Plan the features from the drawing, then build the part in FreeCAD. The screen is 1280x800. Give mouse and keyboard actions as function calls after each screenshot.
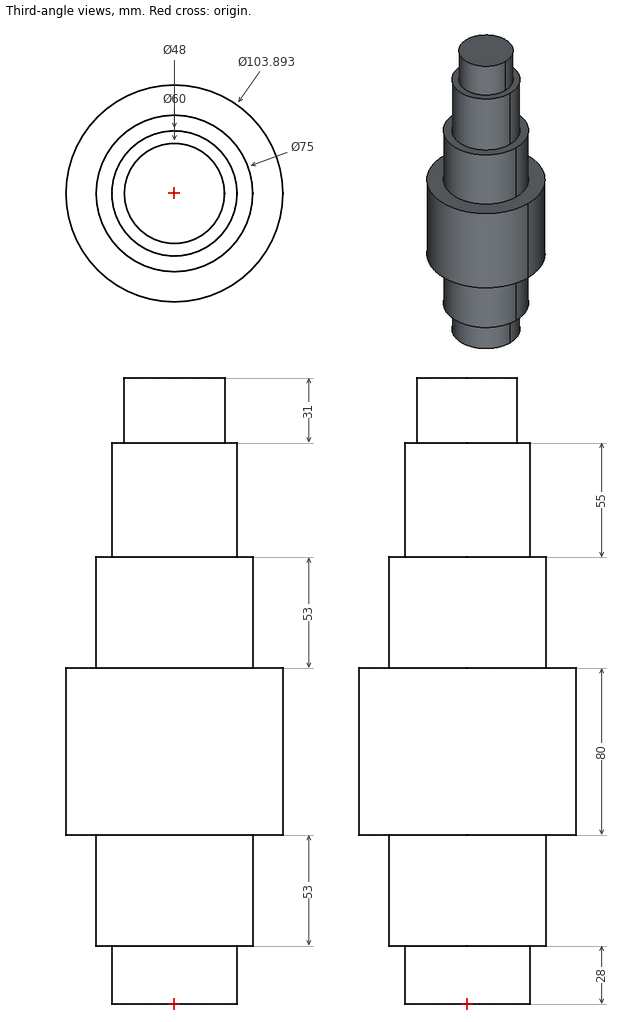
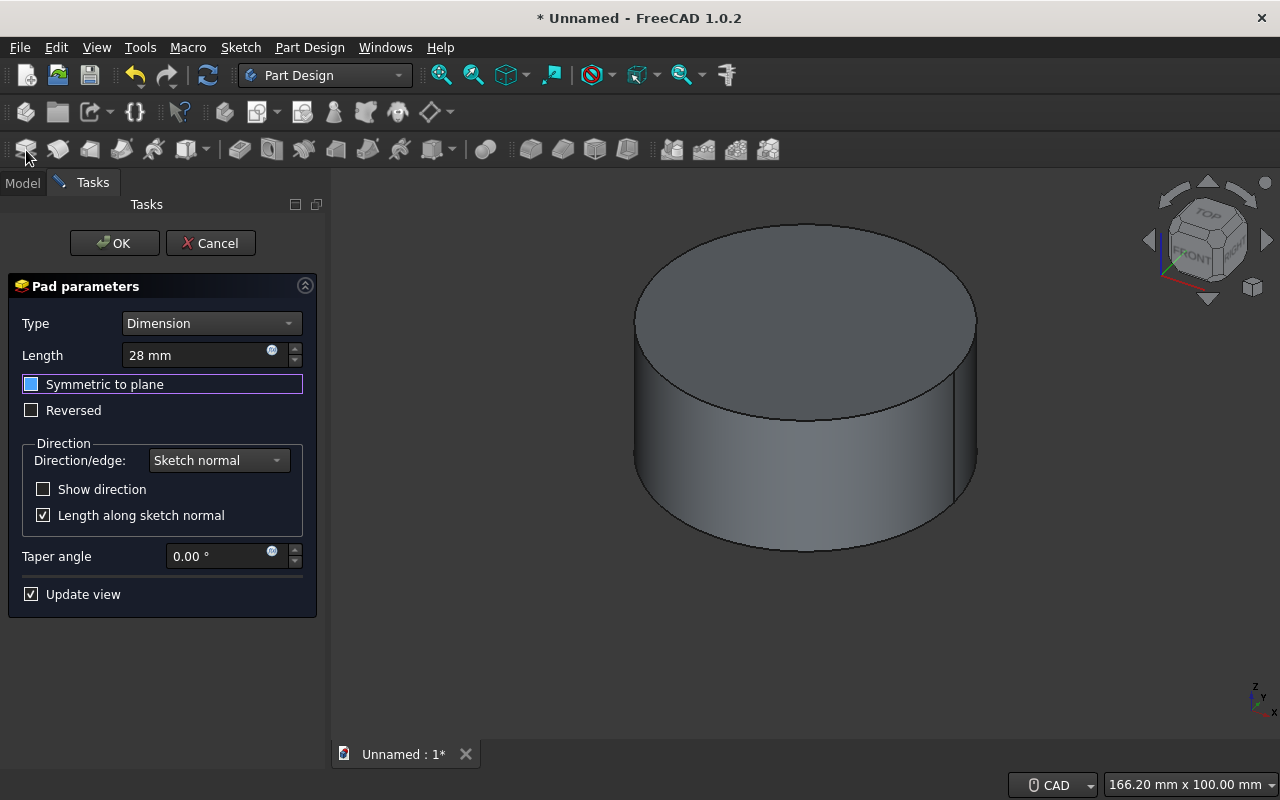
click(115, 243)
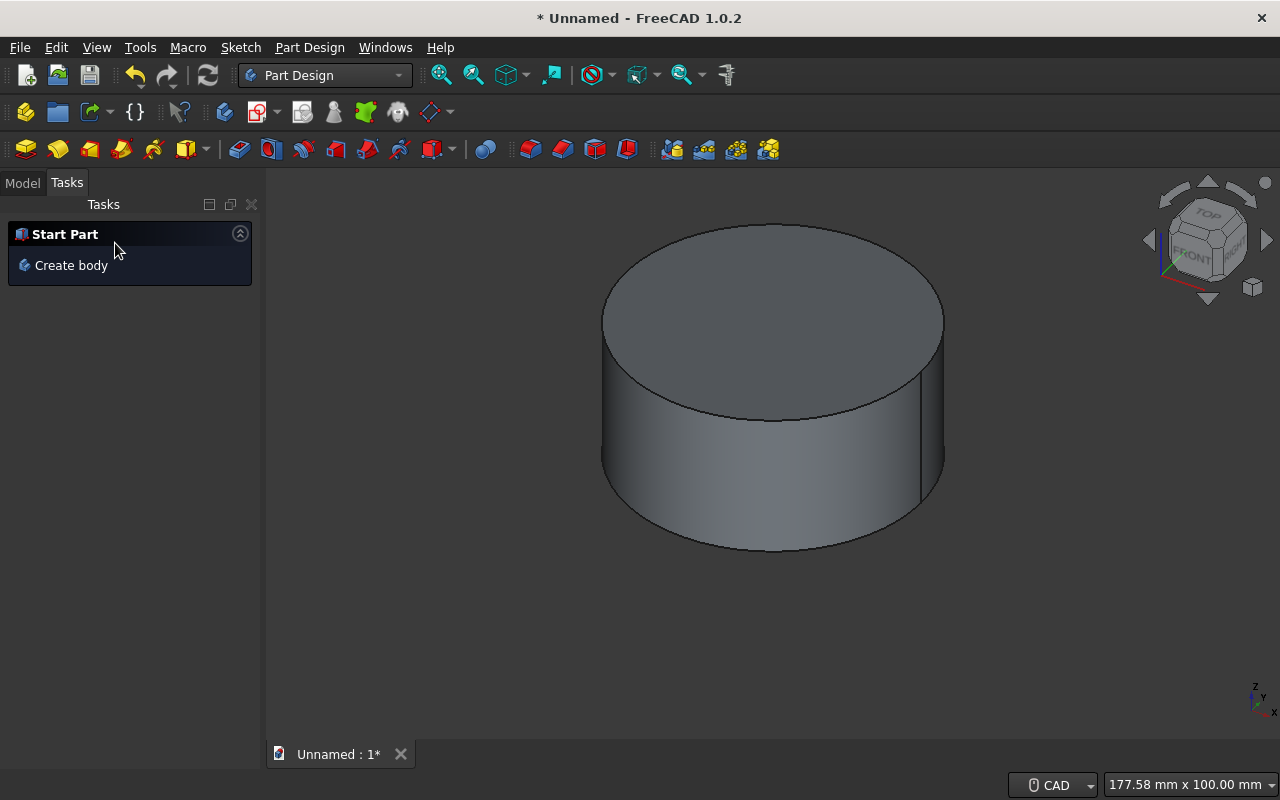
click(773, 322)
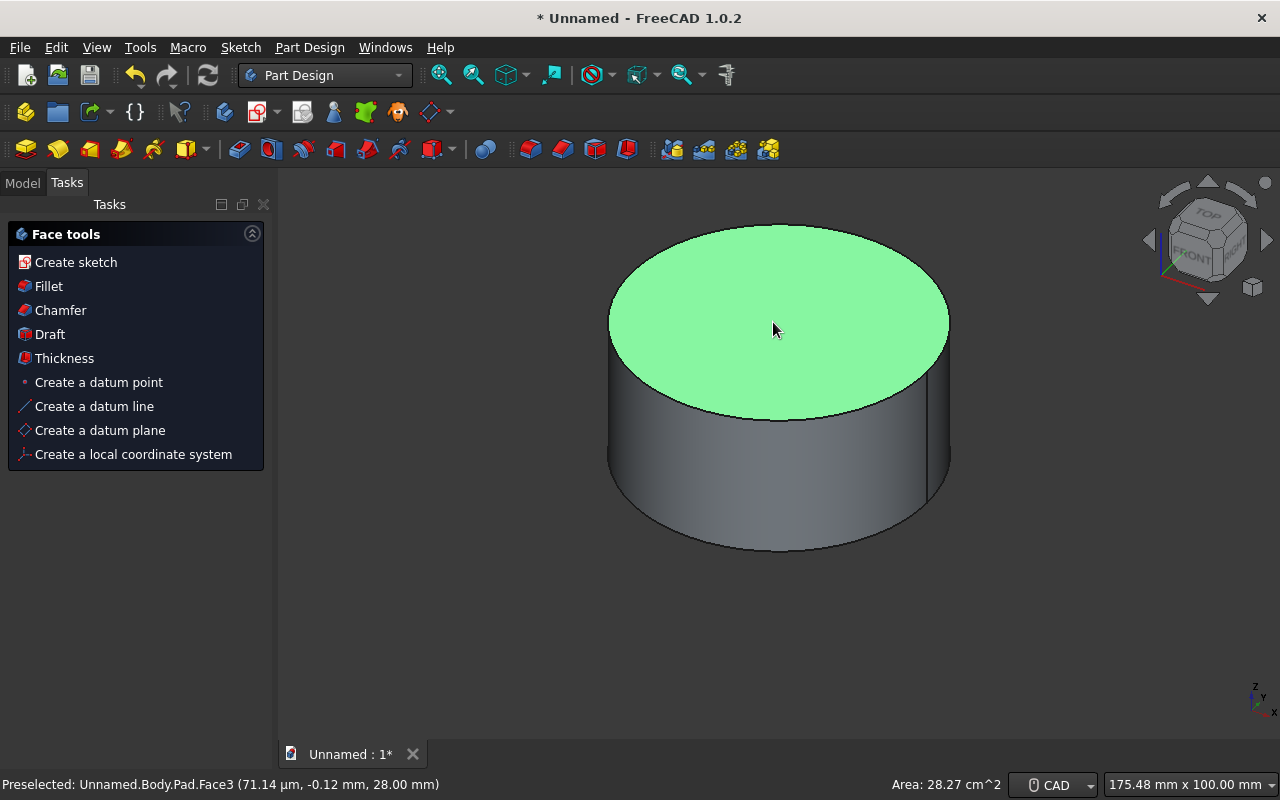
click(258, 112)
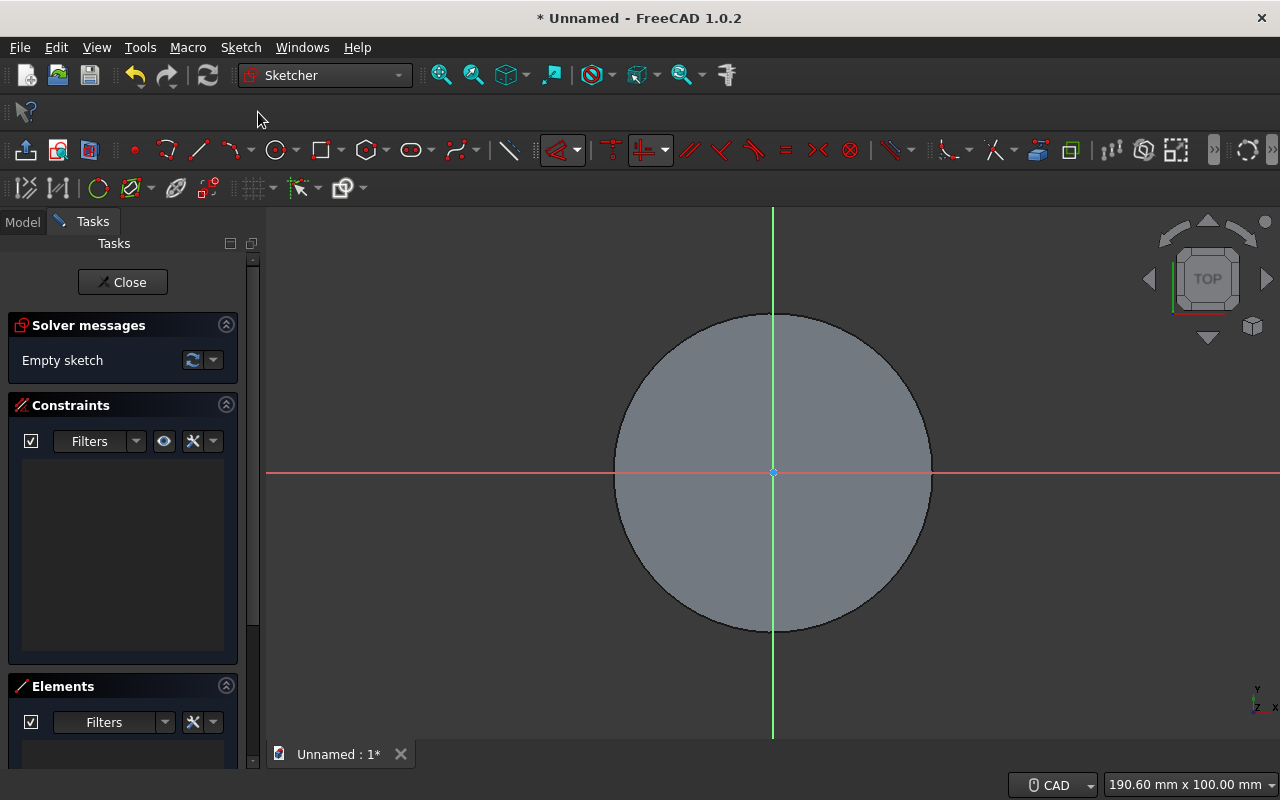
click(276, 150)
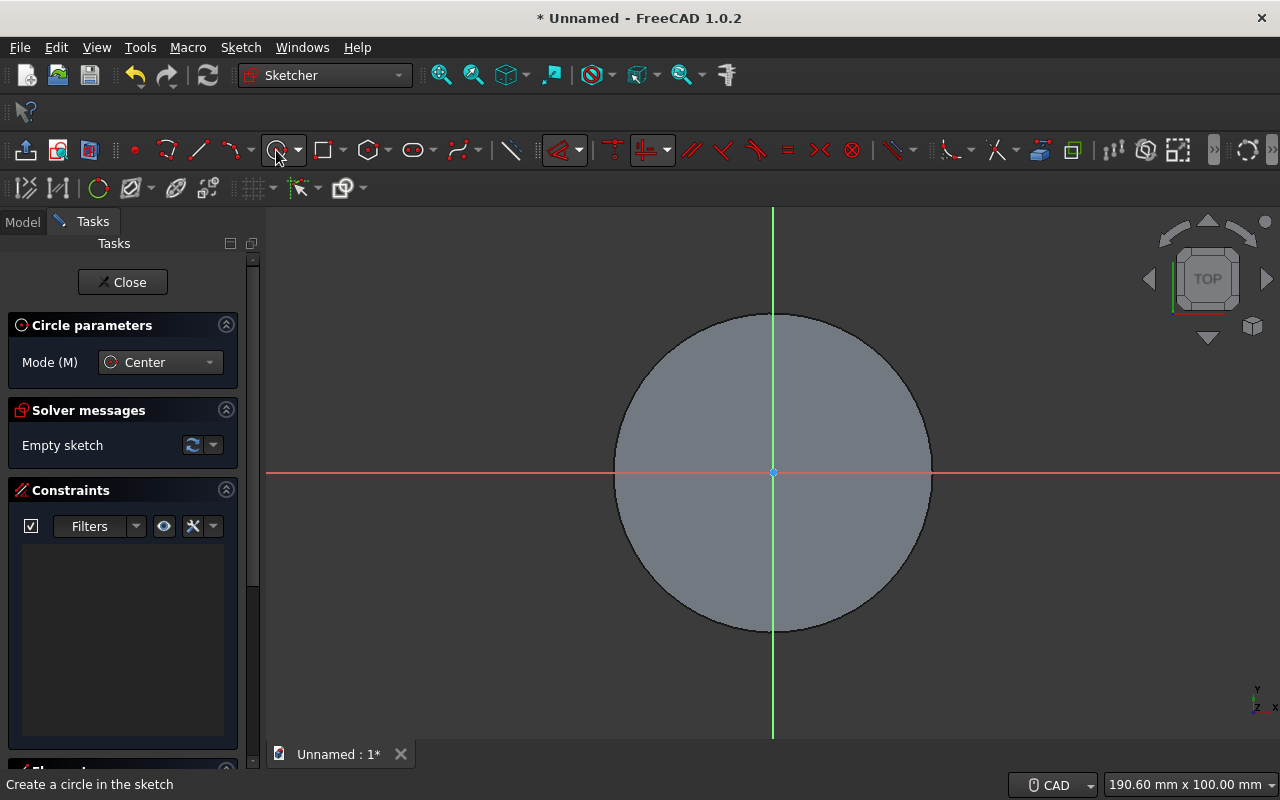
click(773, 473)
move(914, 332)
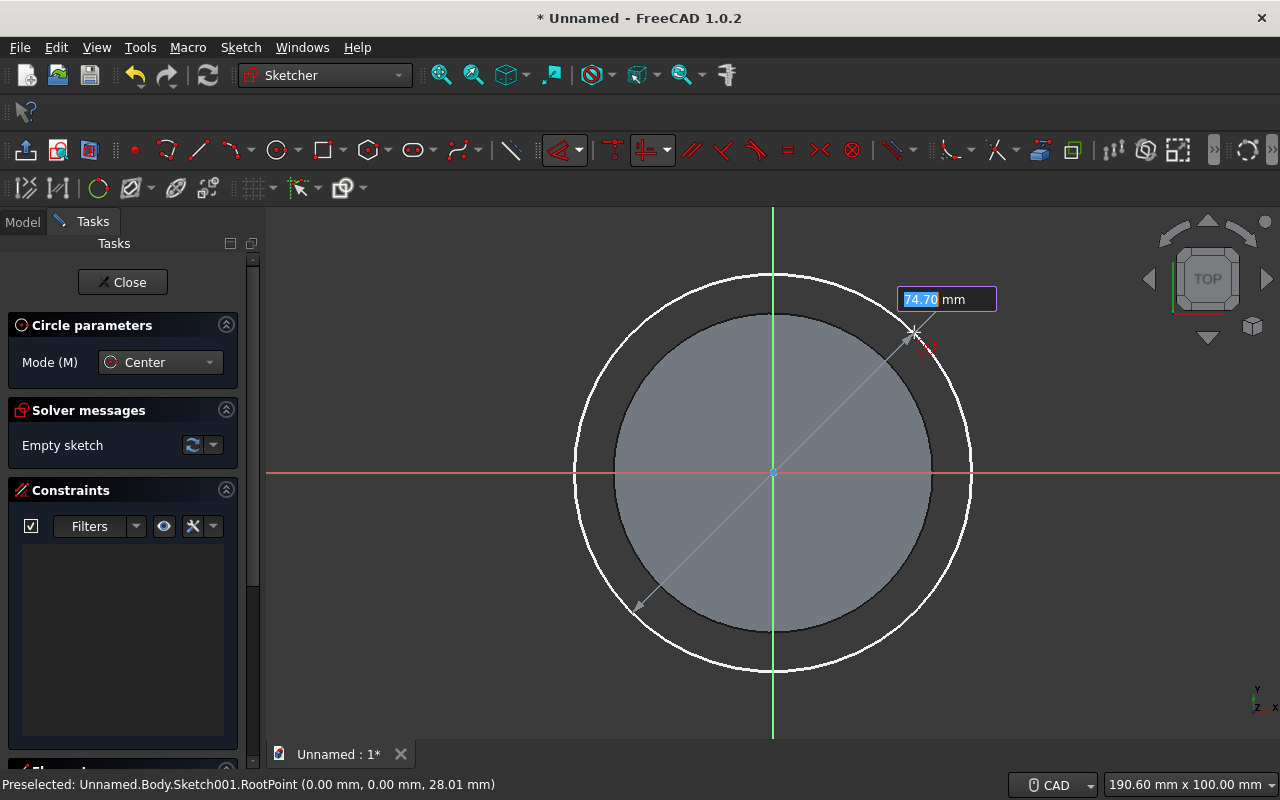
text(75)
key(Return)
key(Escape)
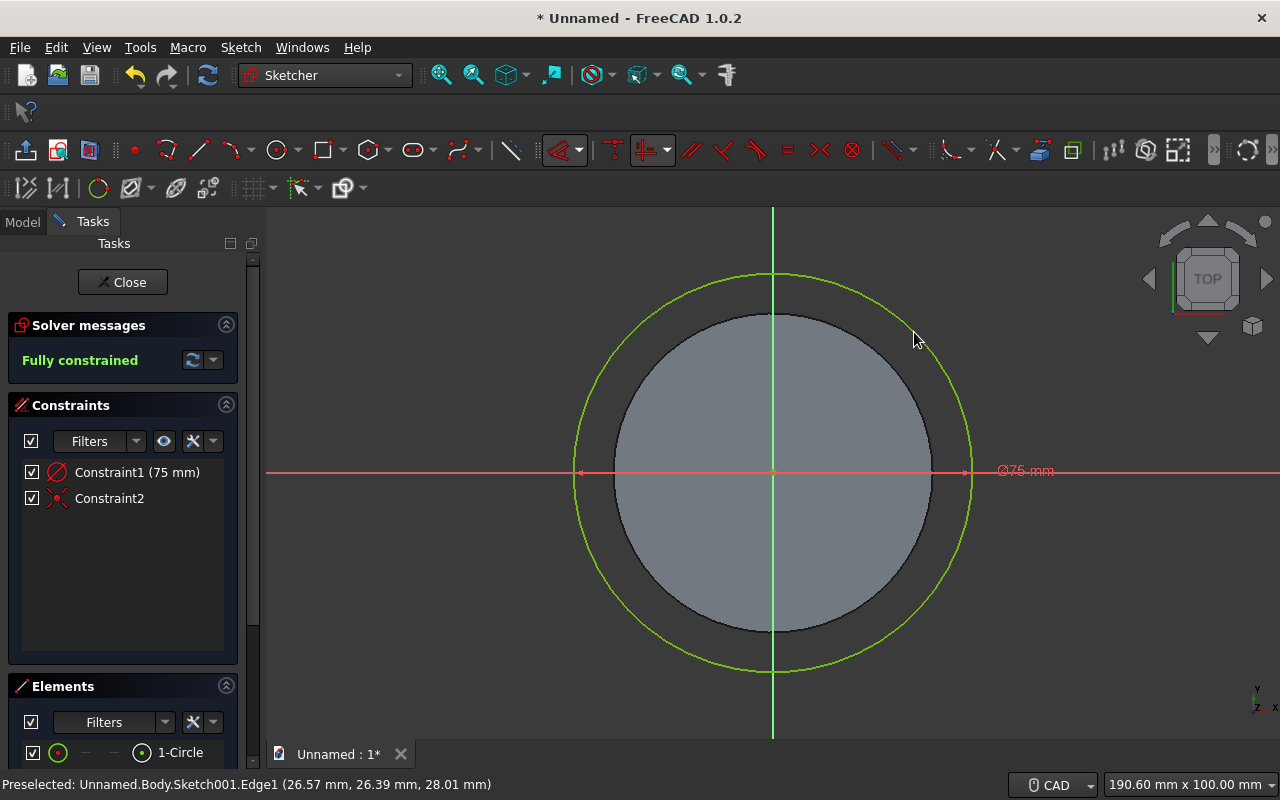
click(123, 282)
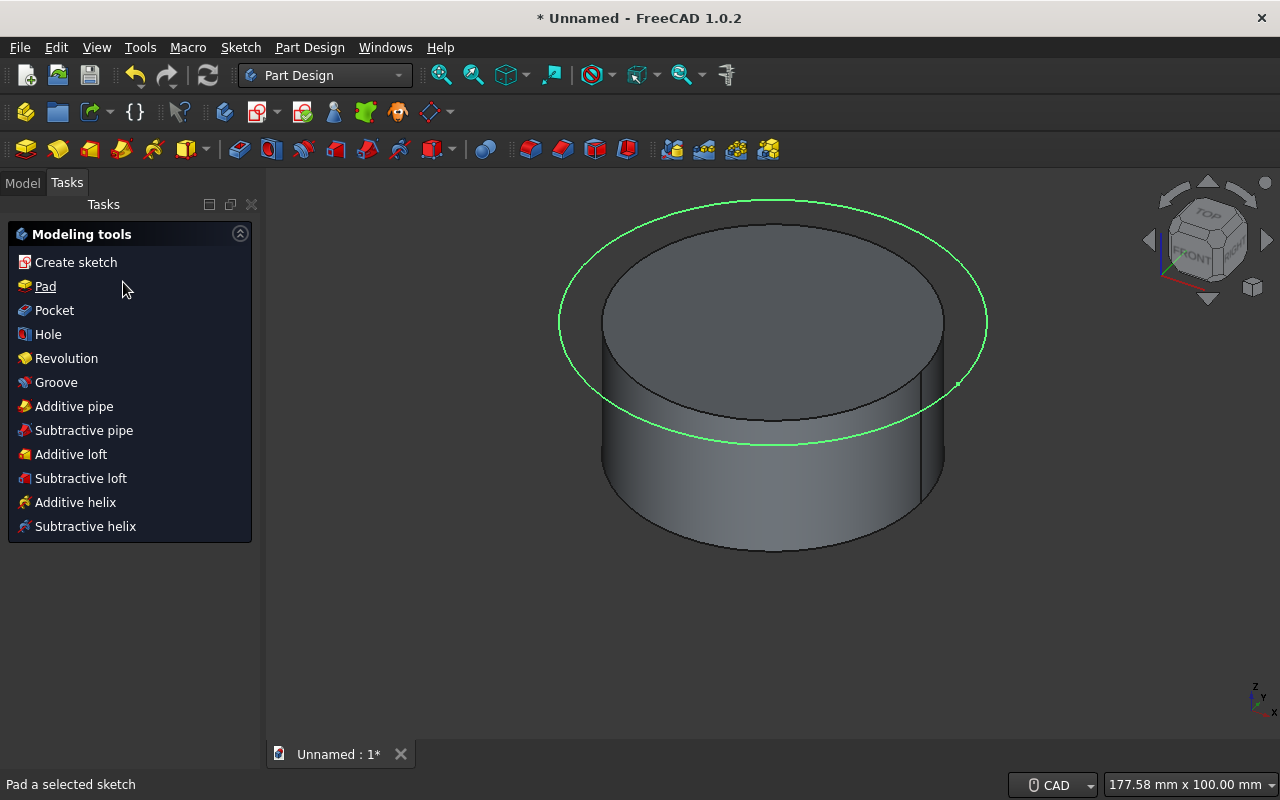
click(26, 150)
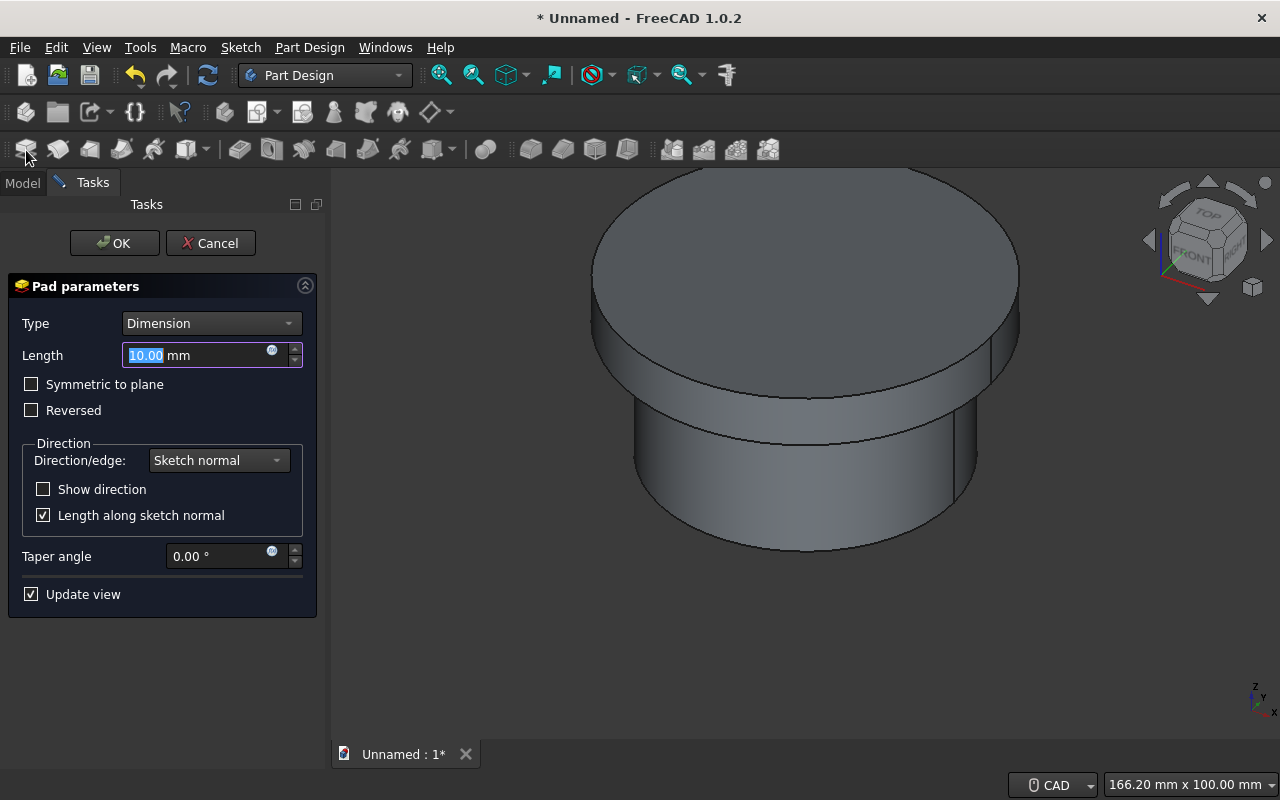
text(53)
key(Tab)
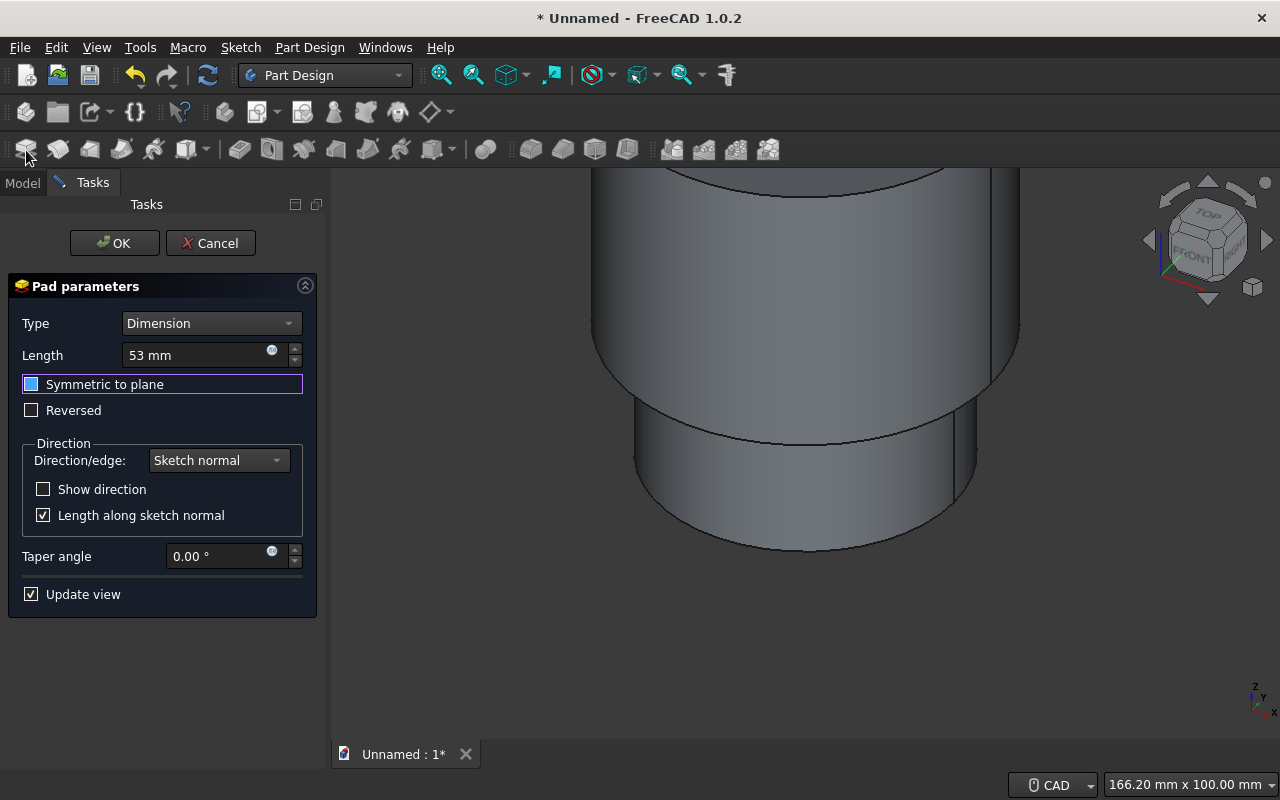
click(115, 243)